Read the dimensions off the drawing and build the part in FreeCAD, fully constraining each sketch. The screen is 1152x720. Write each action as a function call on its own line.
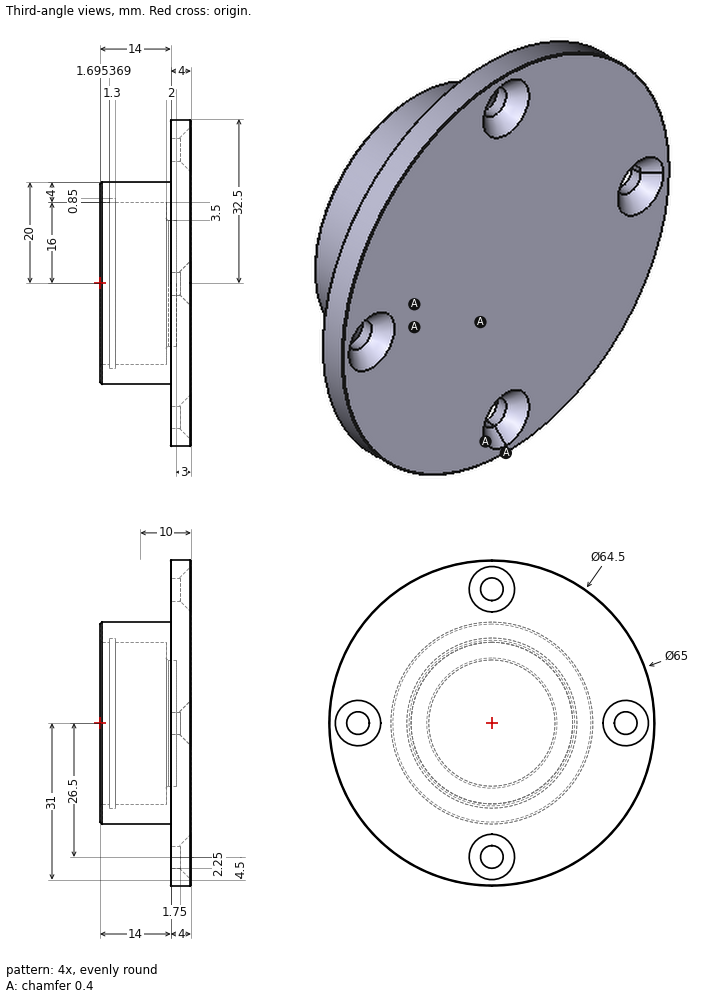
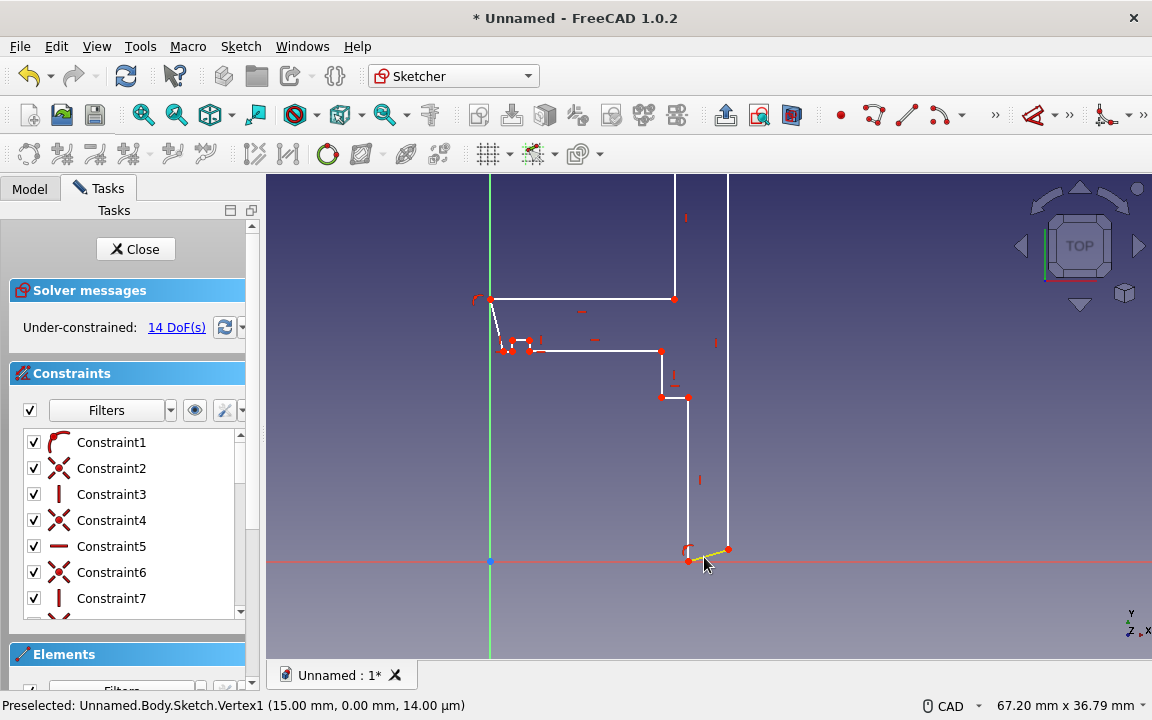
click(704, 557)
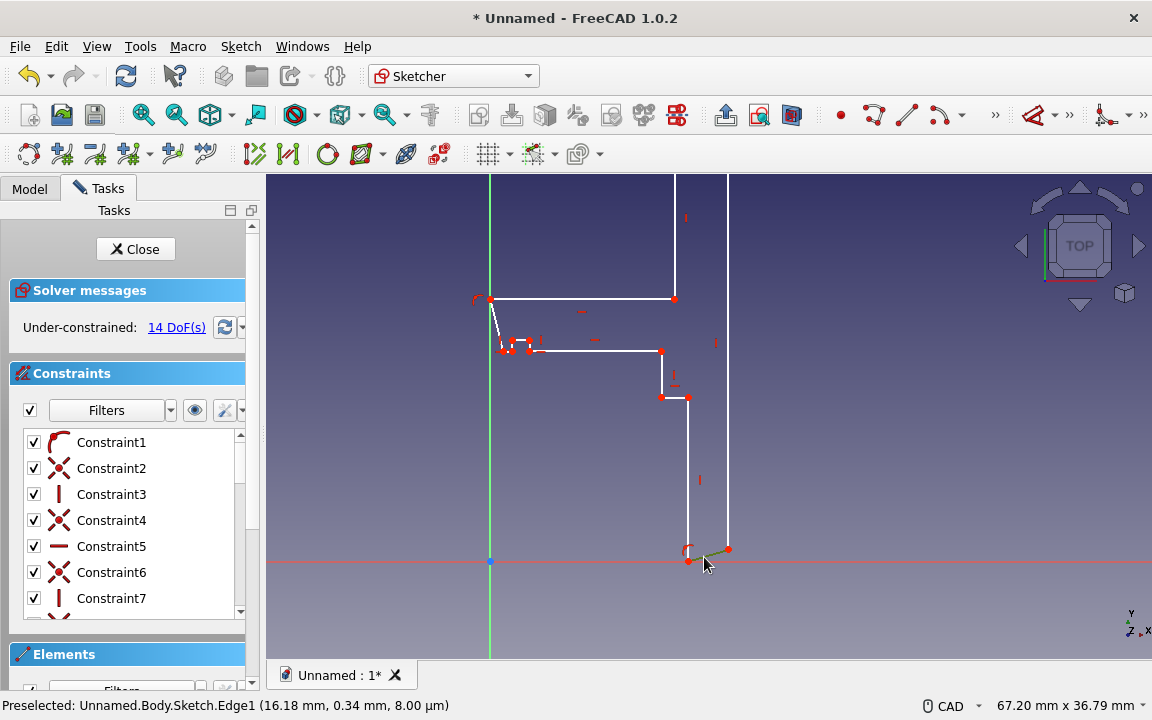
key(h)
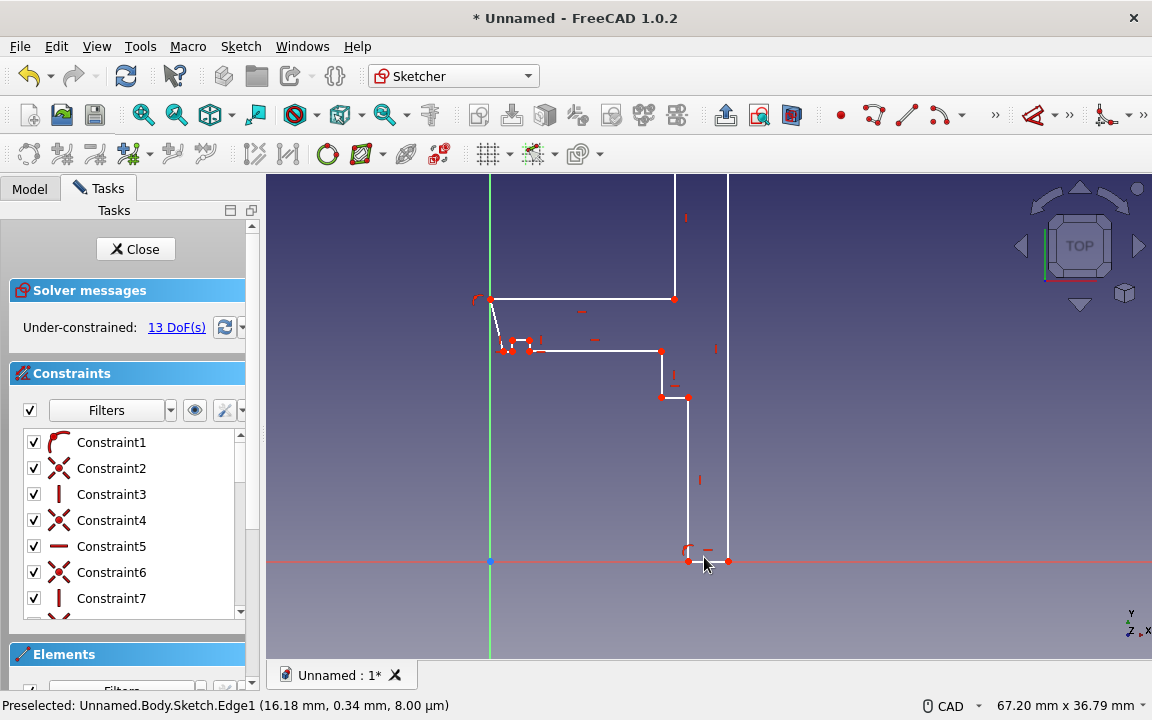
click(494, 315)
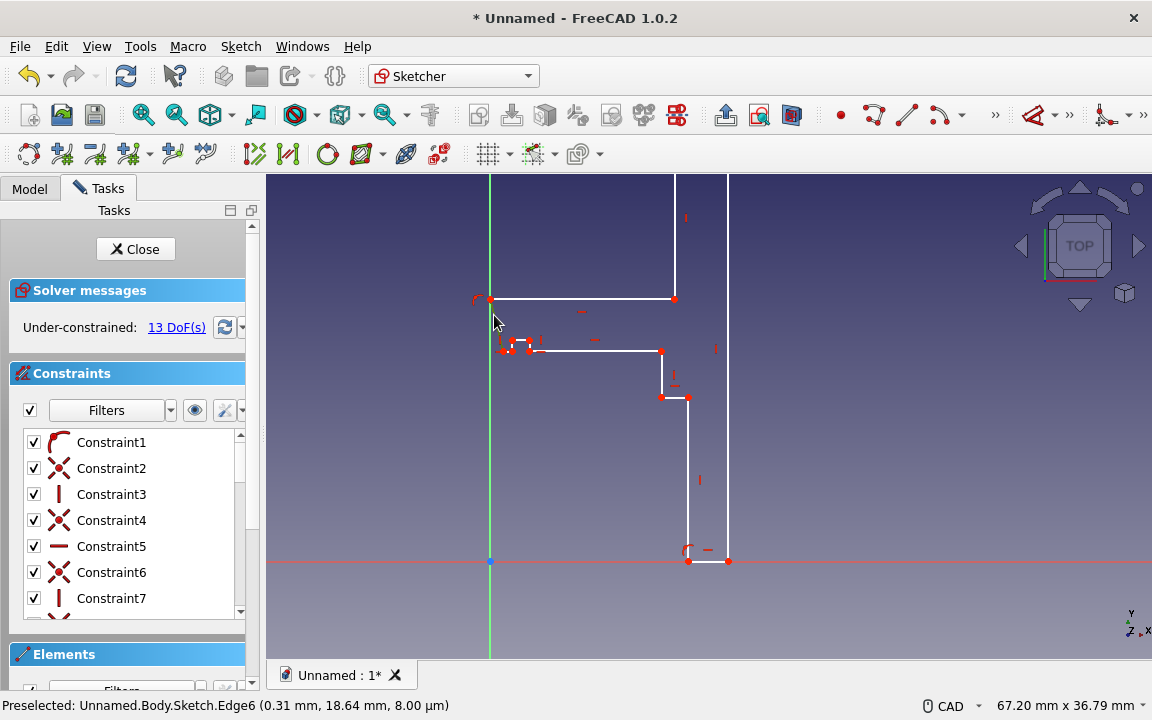
key(v)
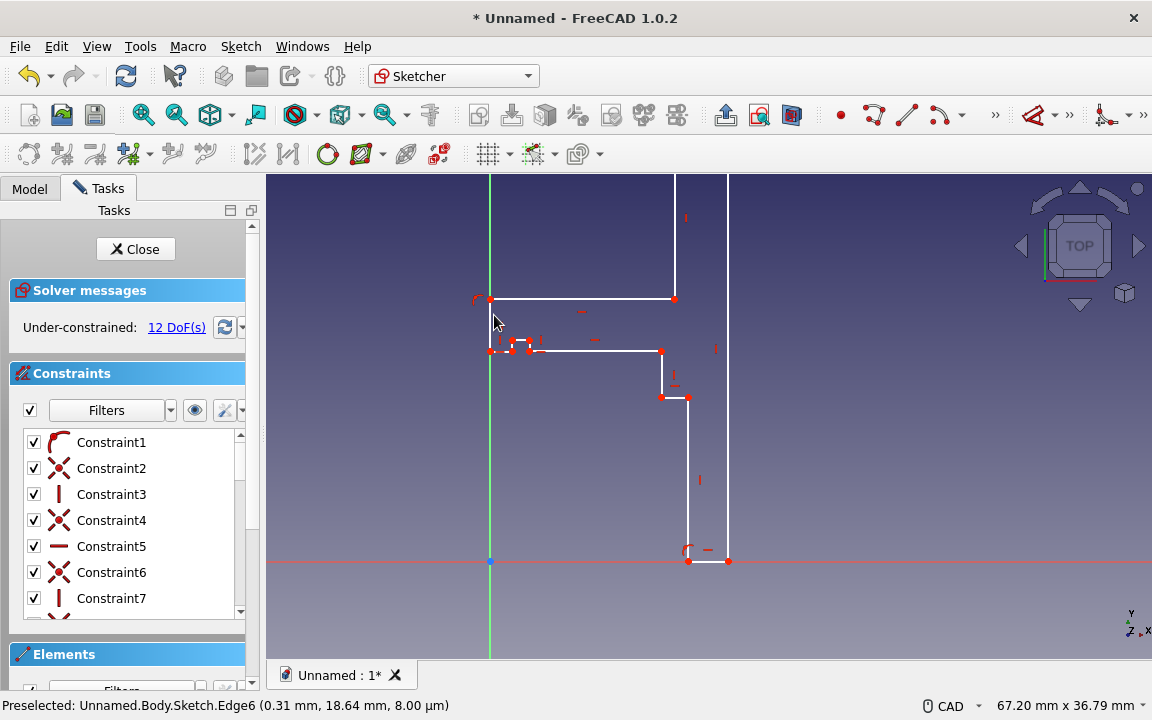
click(700, 562)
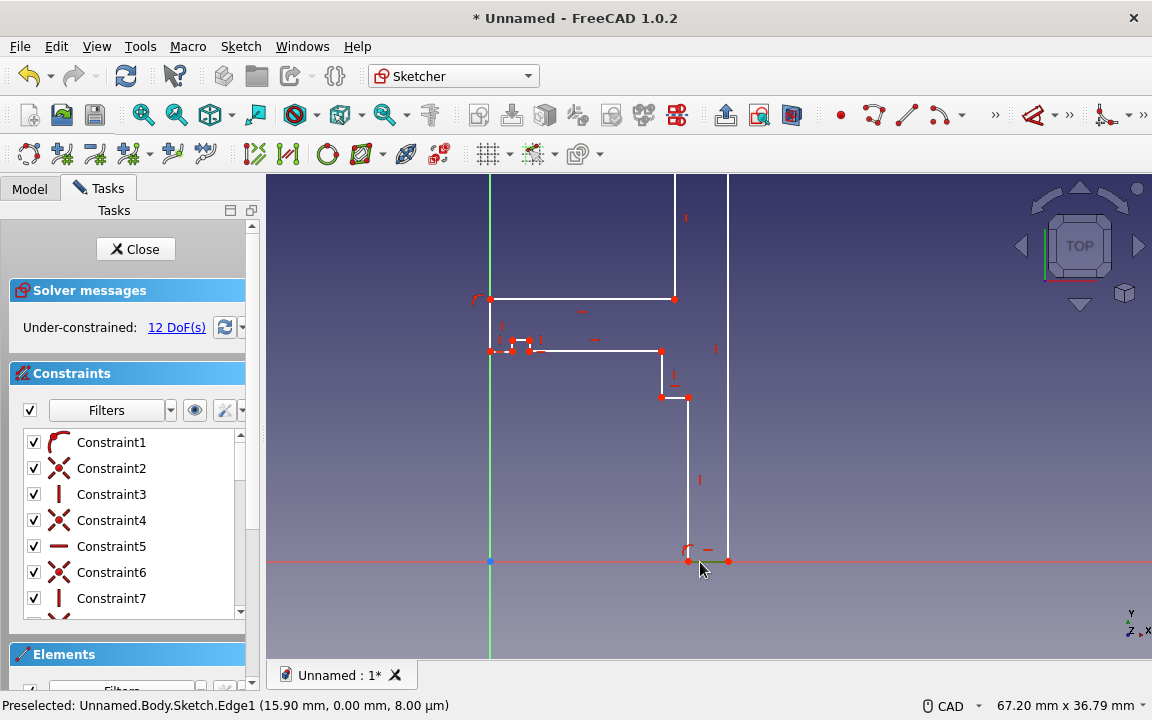
click(1054, 116)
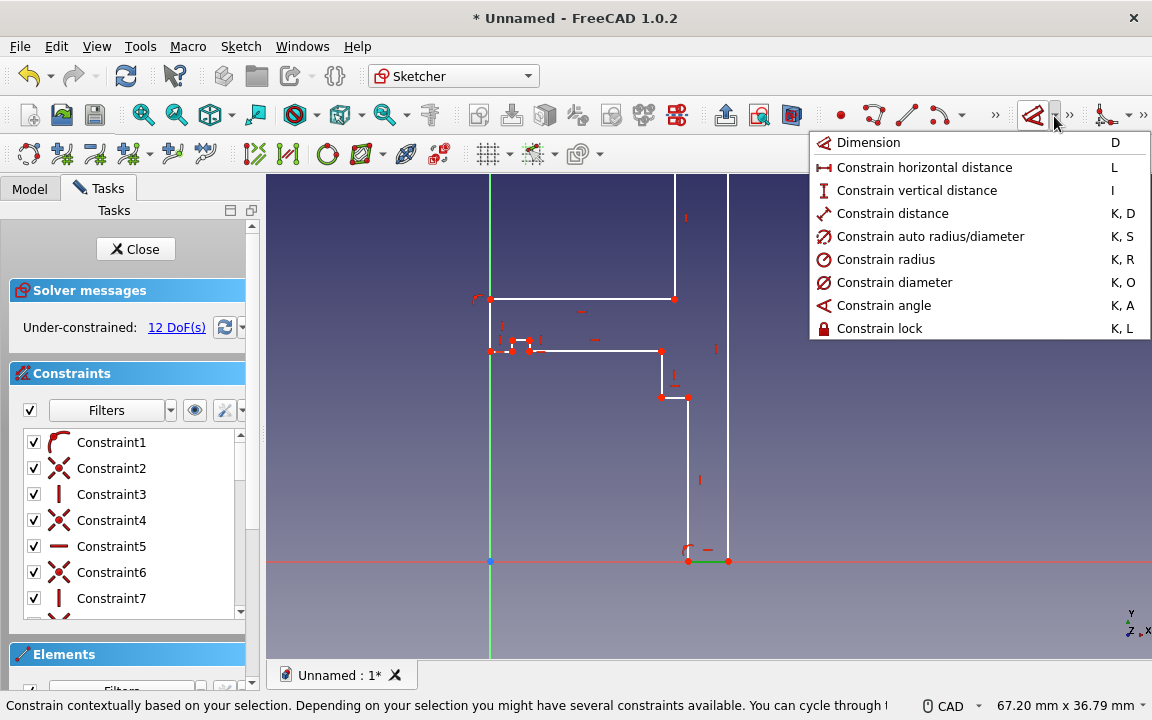
click(980, 168)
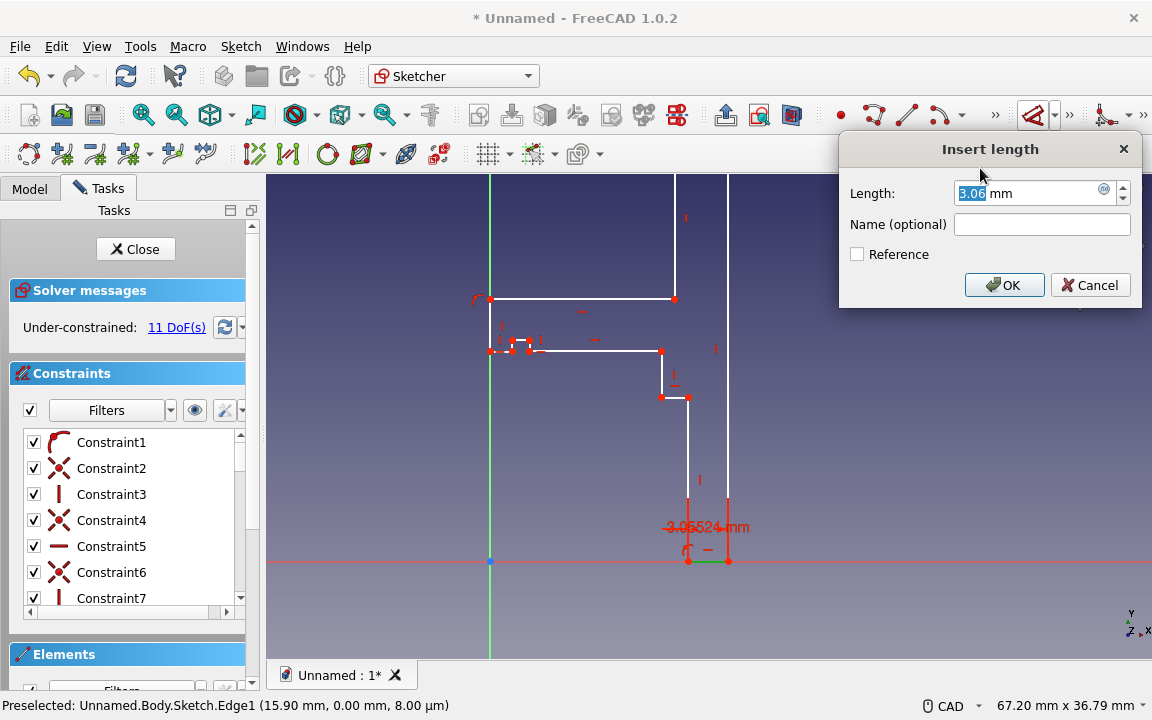
text(3)
key(Return)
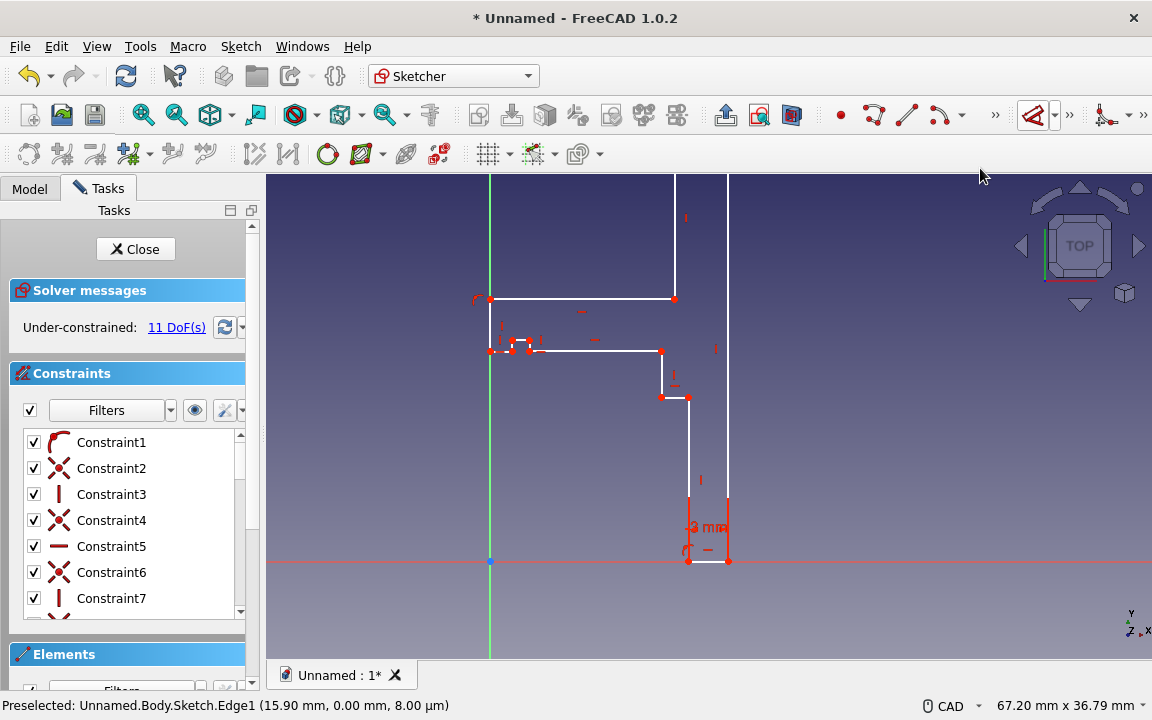
scroll(704, 557, down, 2)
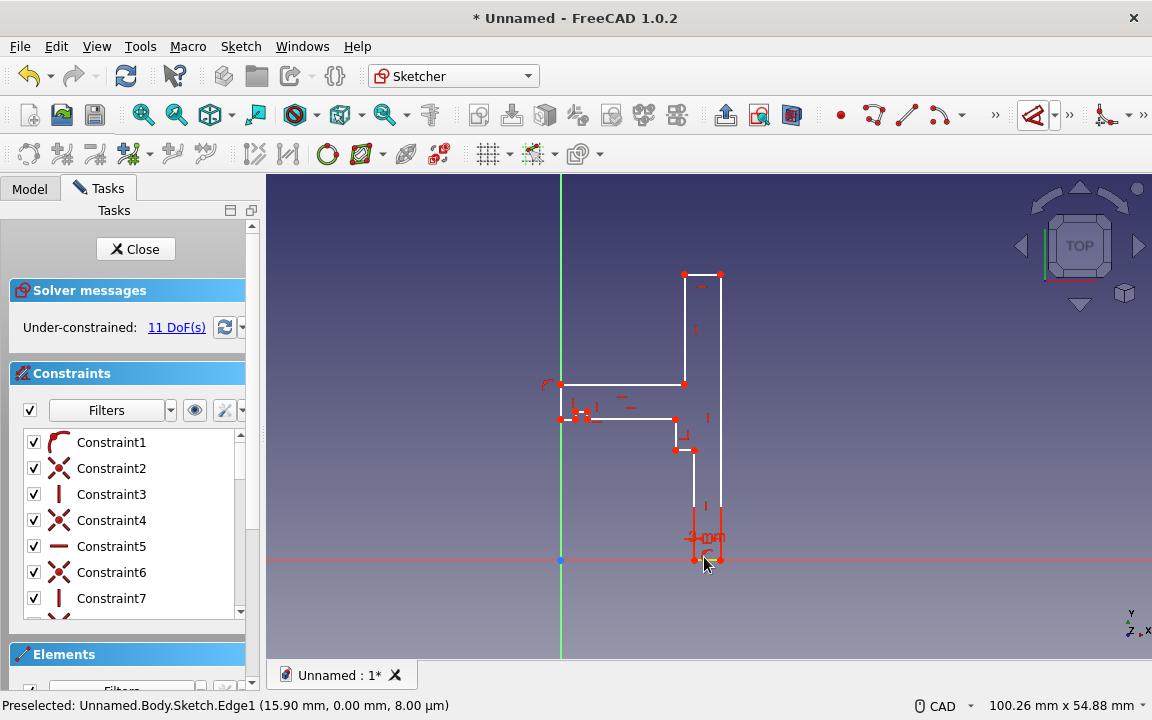
scroll(710, 275, up, 2)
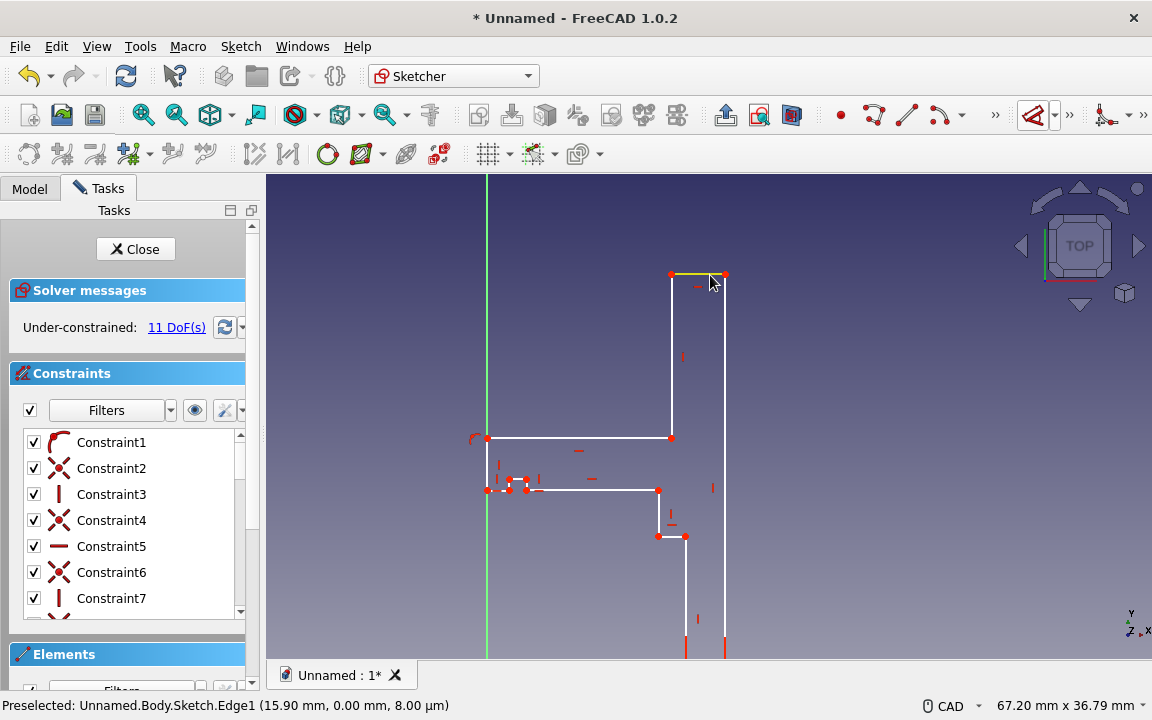
click(709, 274)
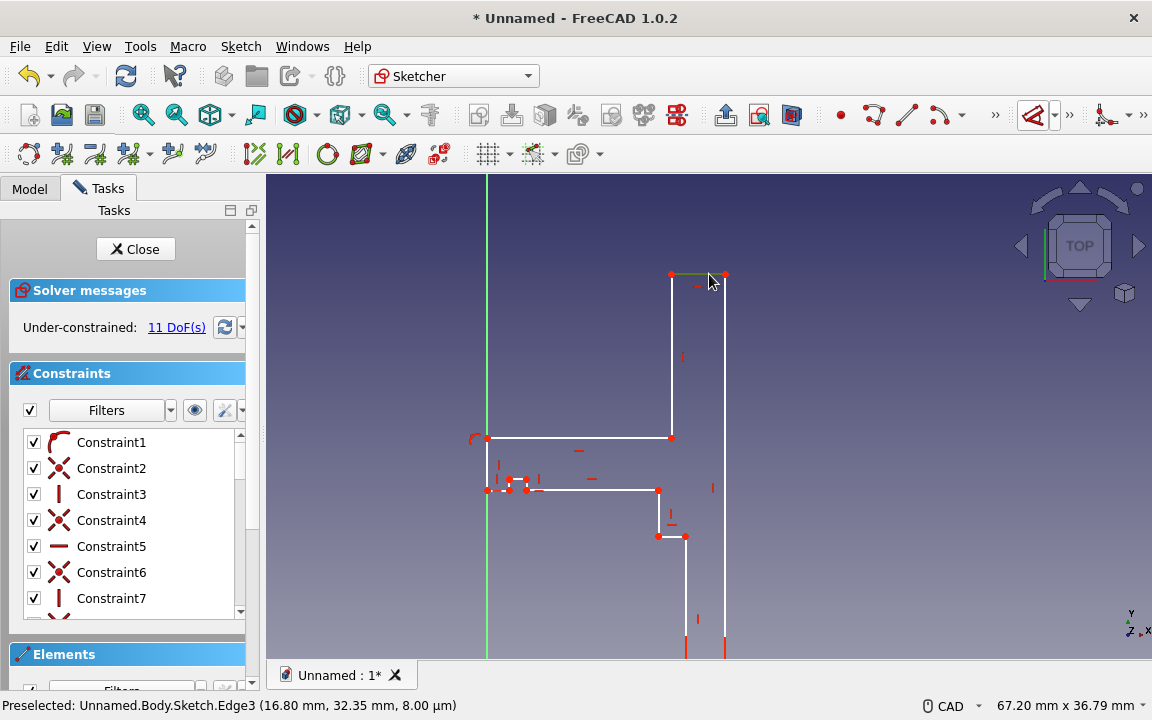
key(l)